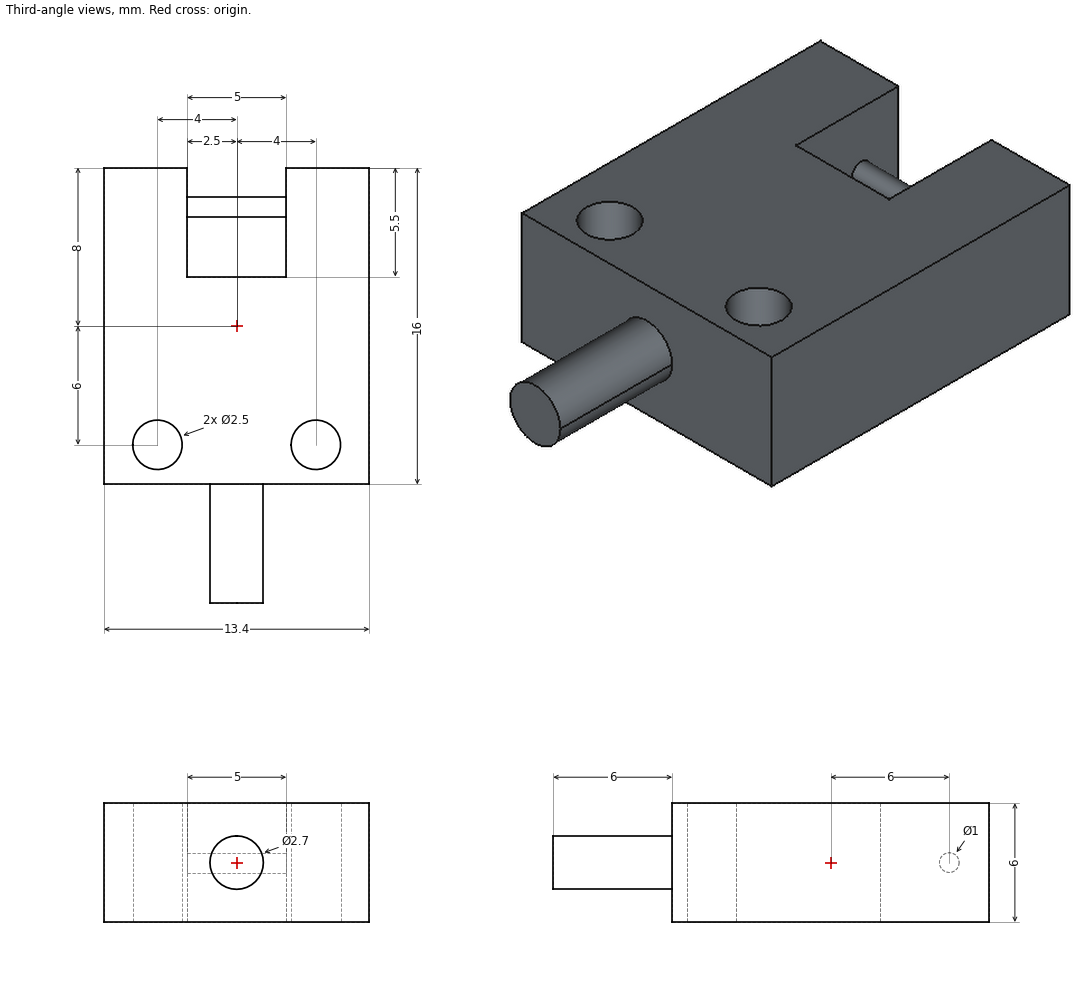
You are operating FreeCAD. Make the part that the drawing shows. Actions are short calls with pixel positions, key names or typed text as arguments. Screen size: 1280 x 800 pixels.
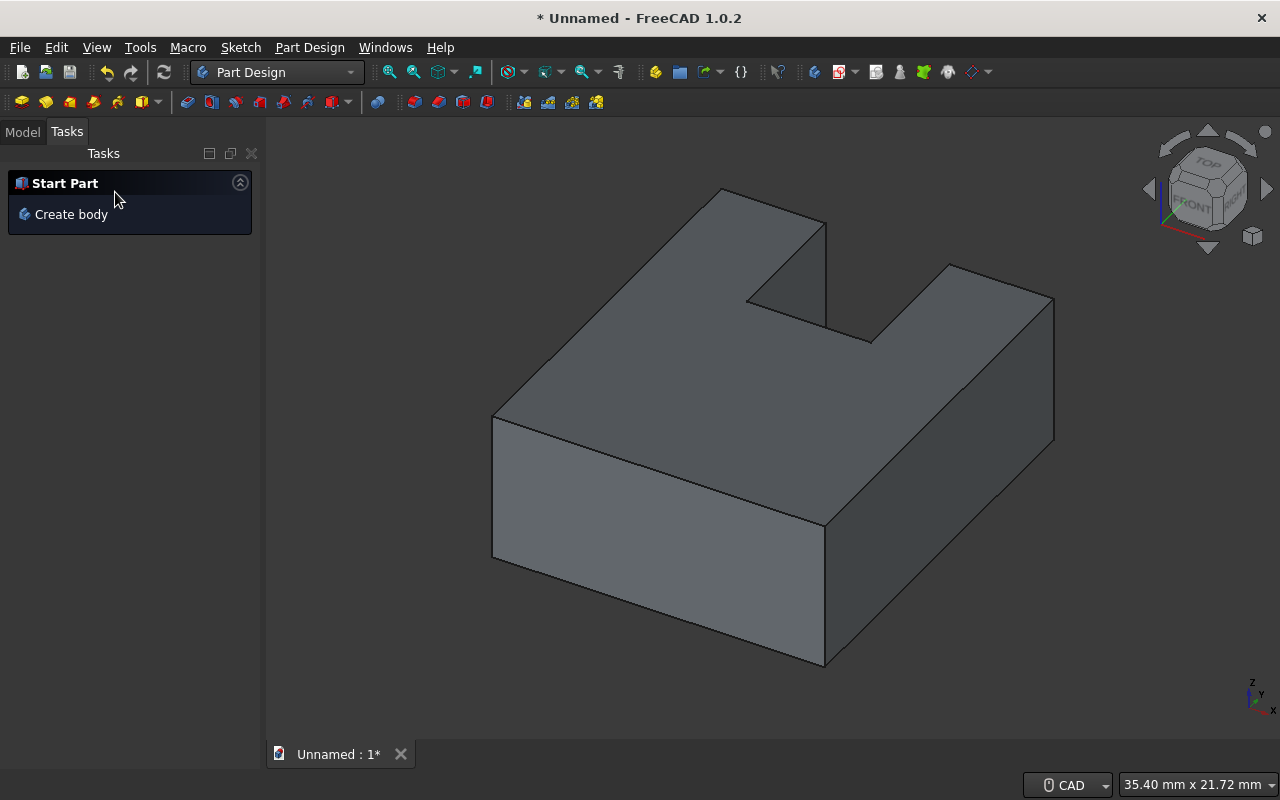
click(706, 557)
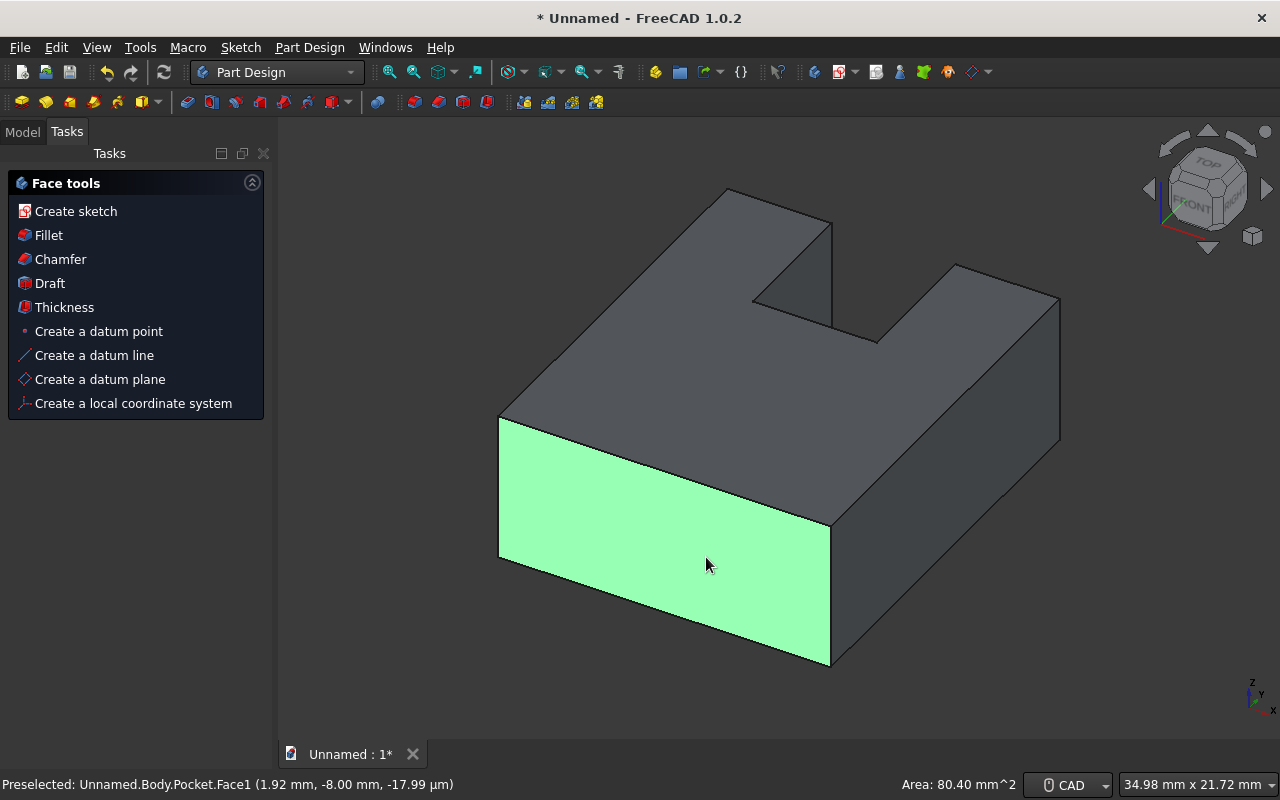
click(840, 72)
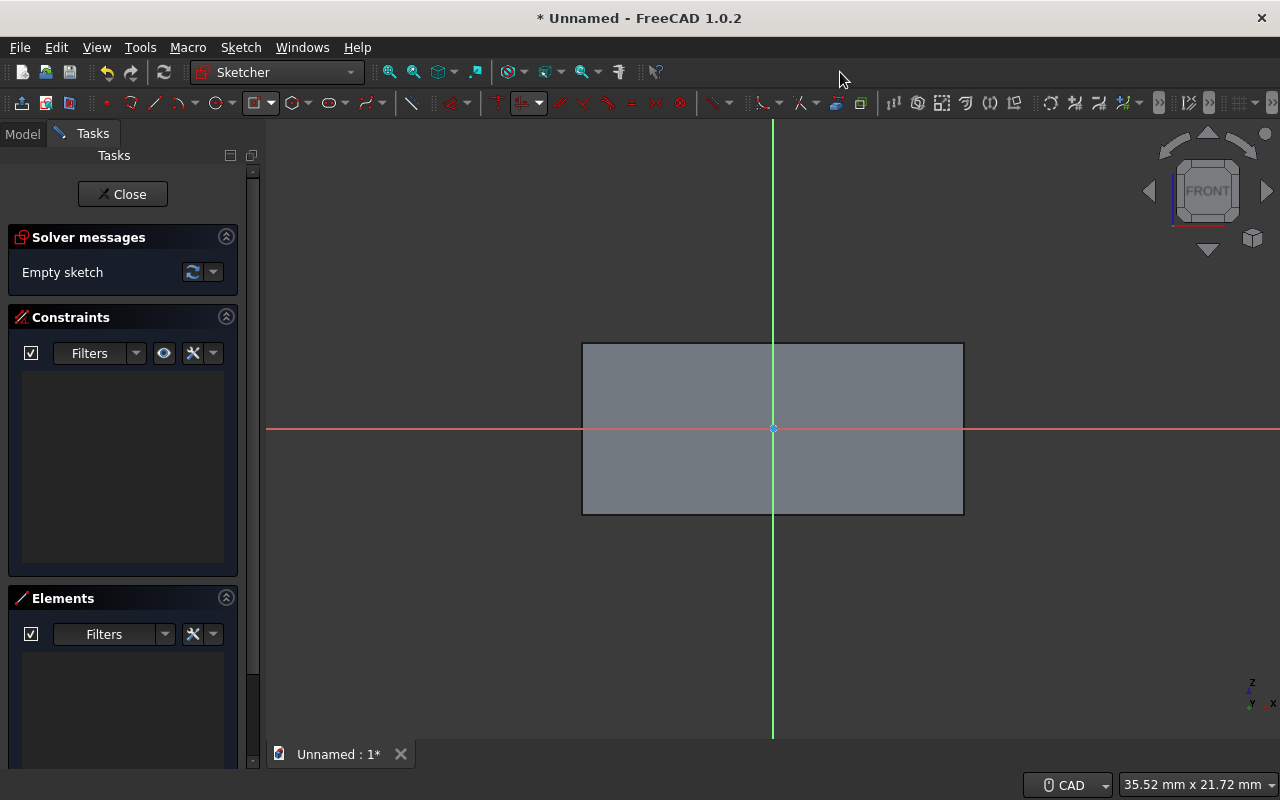
scroll(790, 429, up, 8)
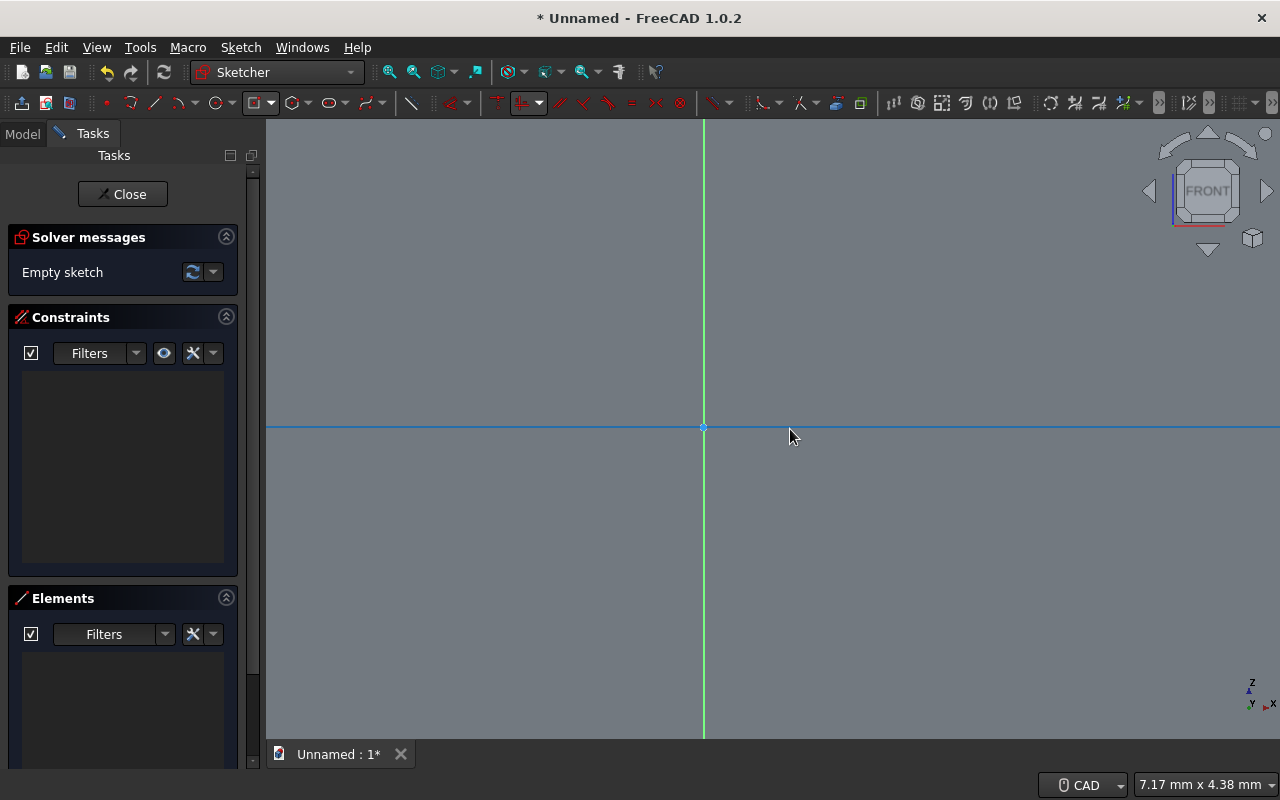
click(216, 104)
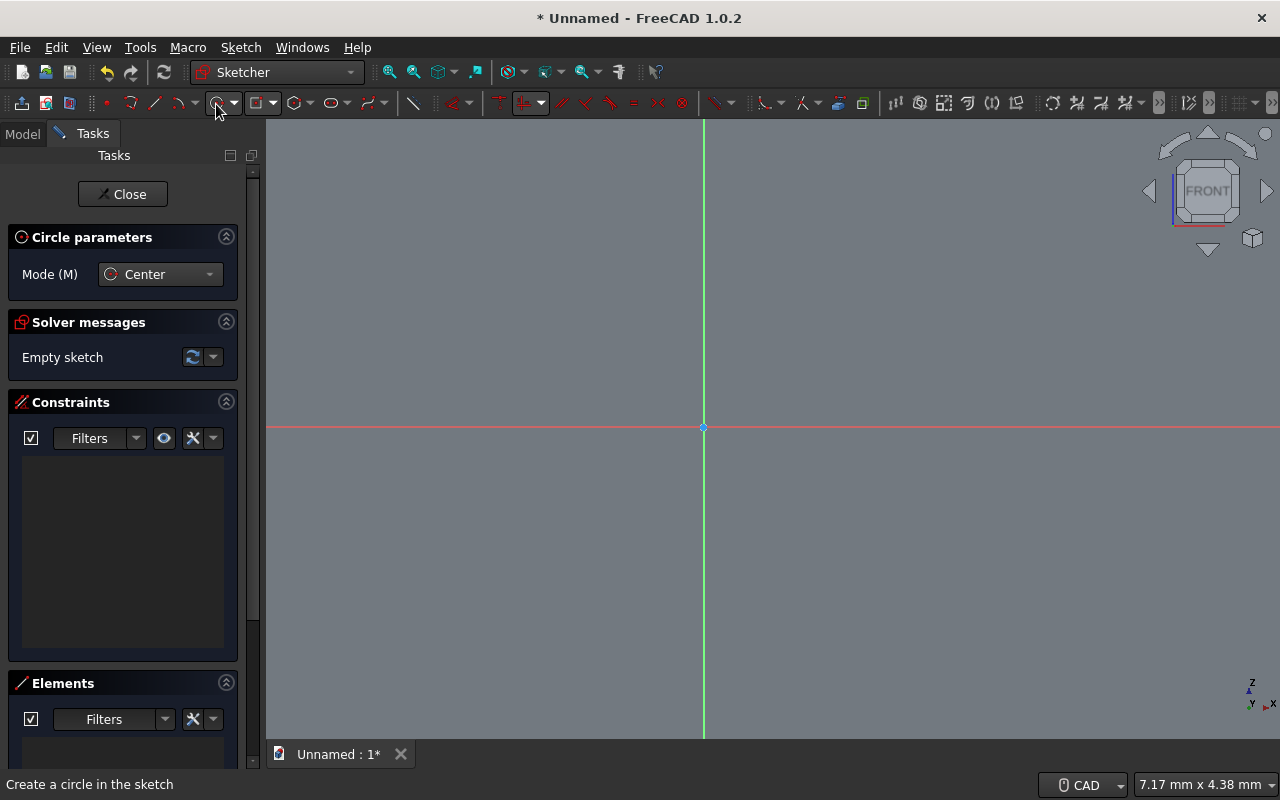
click(704, 427)
move(839, 292)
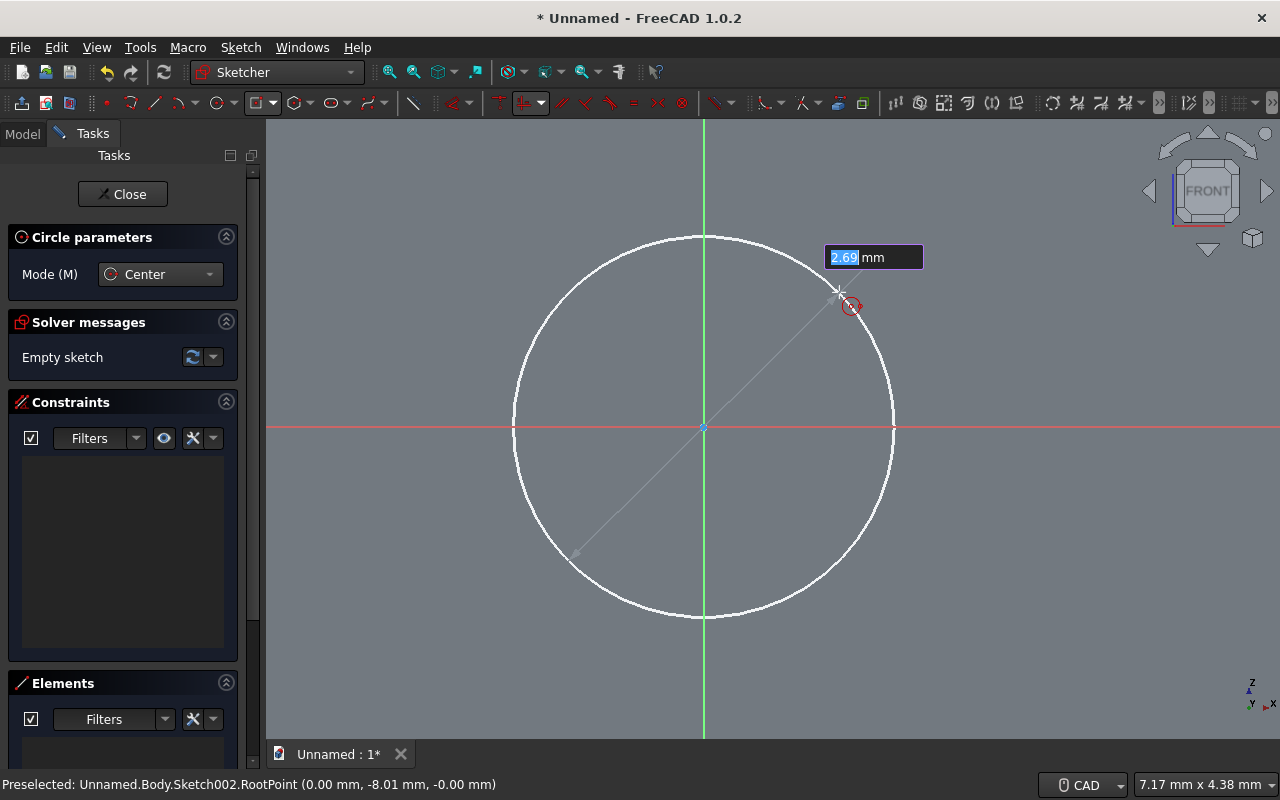
text(2.7)
key(Return)
key(Escape)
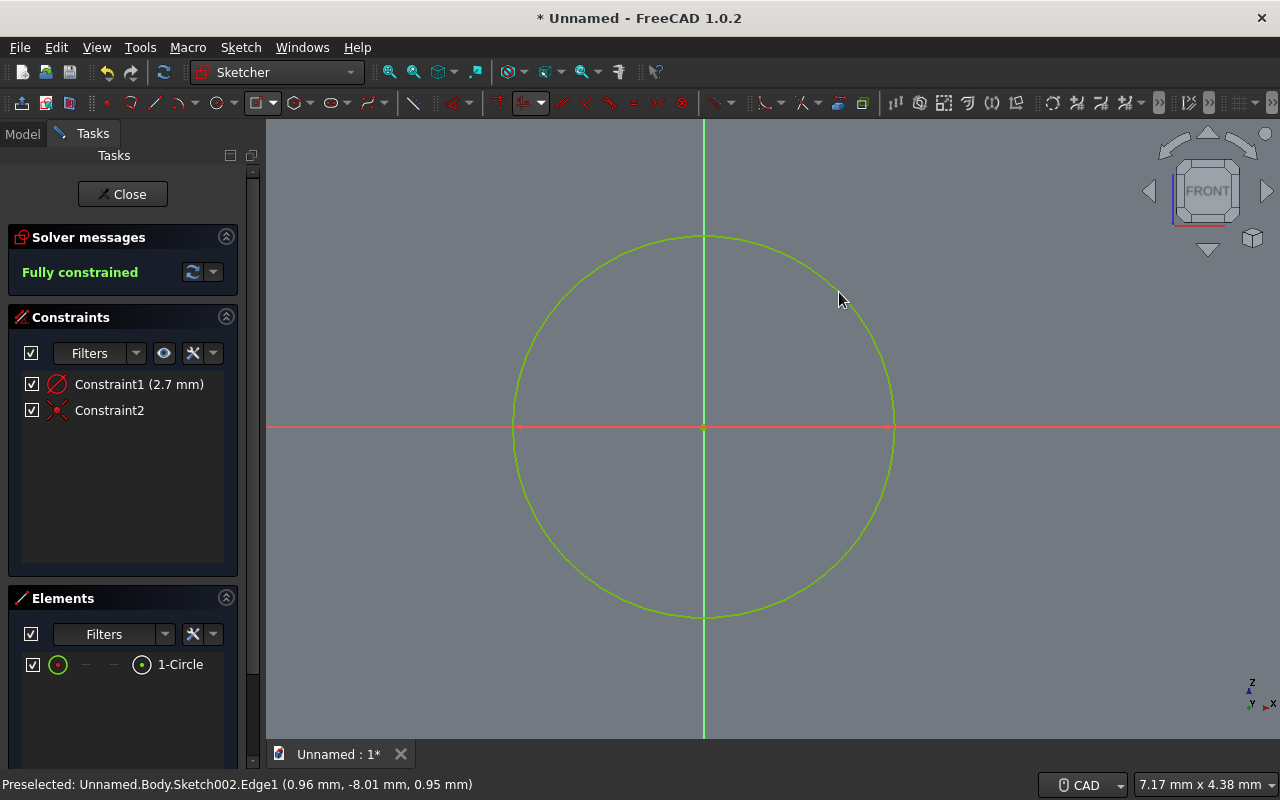
click(123, 194)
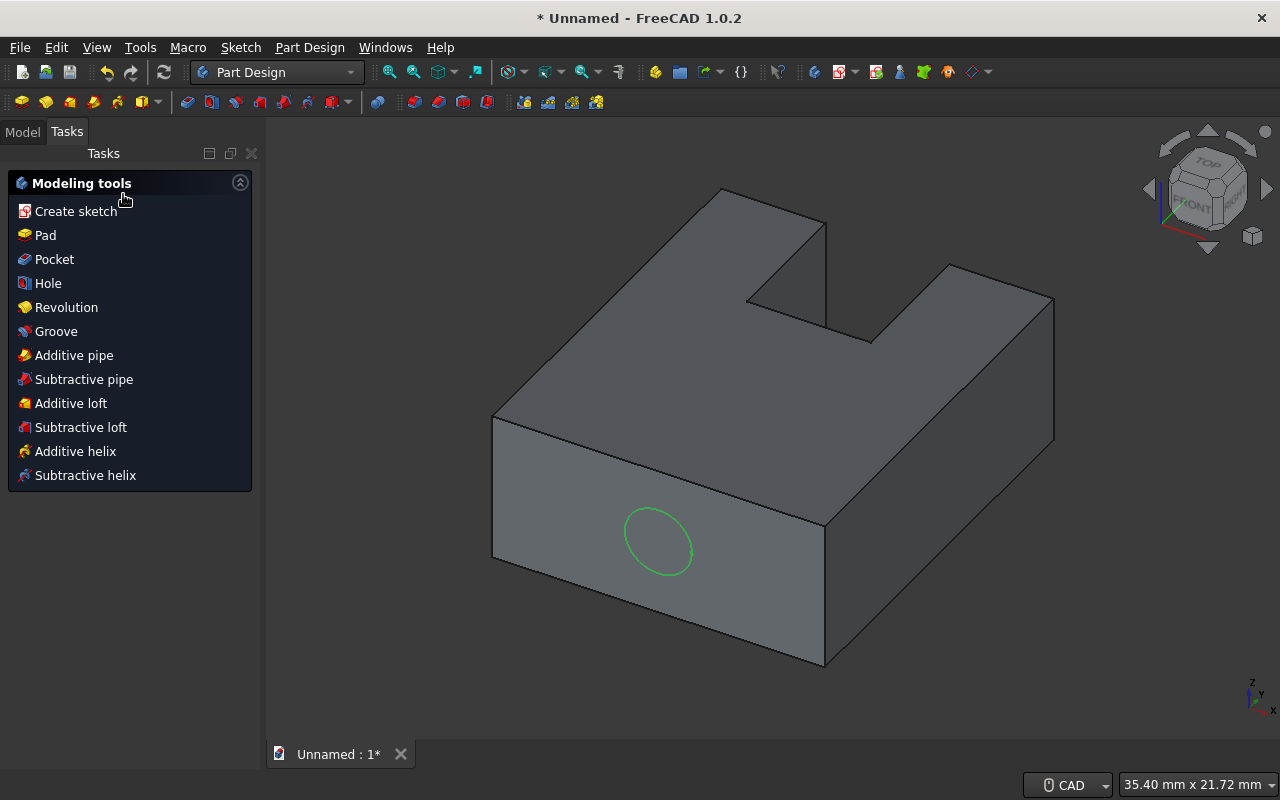
click(22, 102)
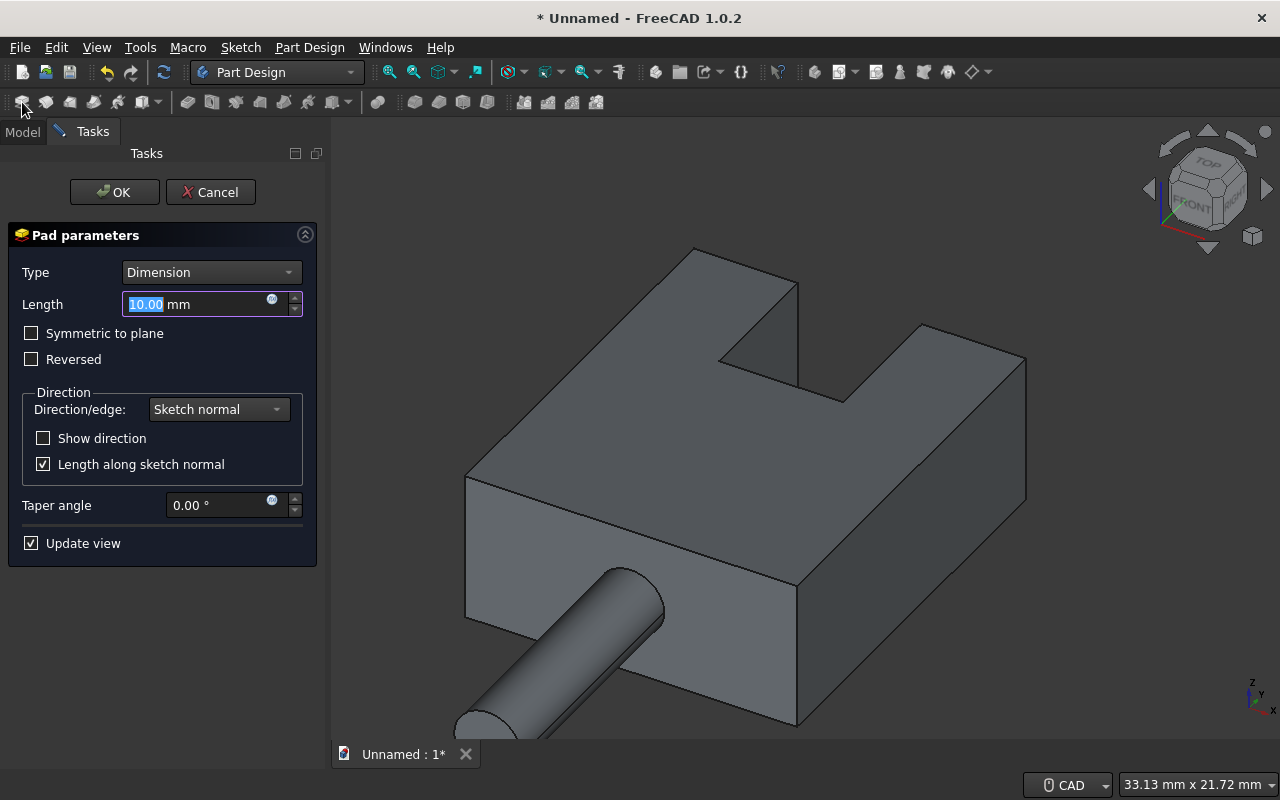
text(6)
key(Tab)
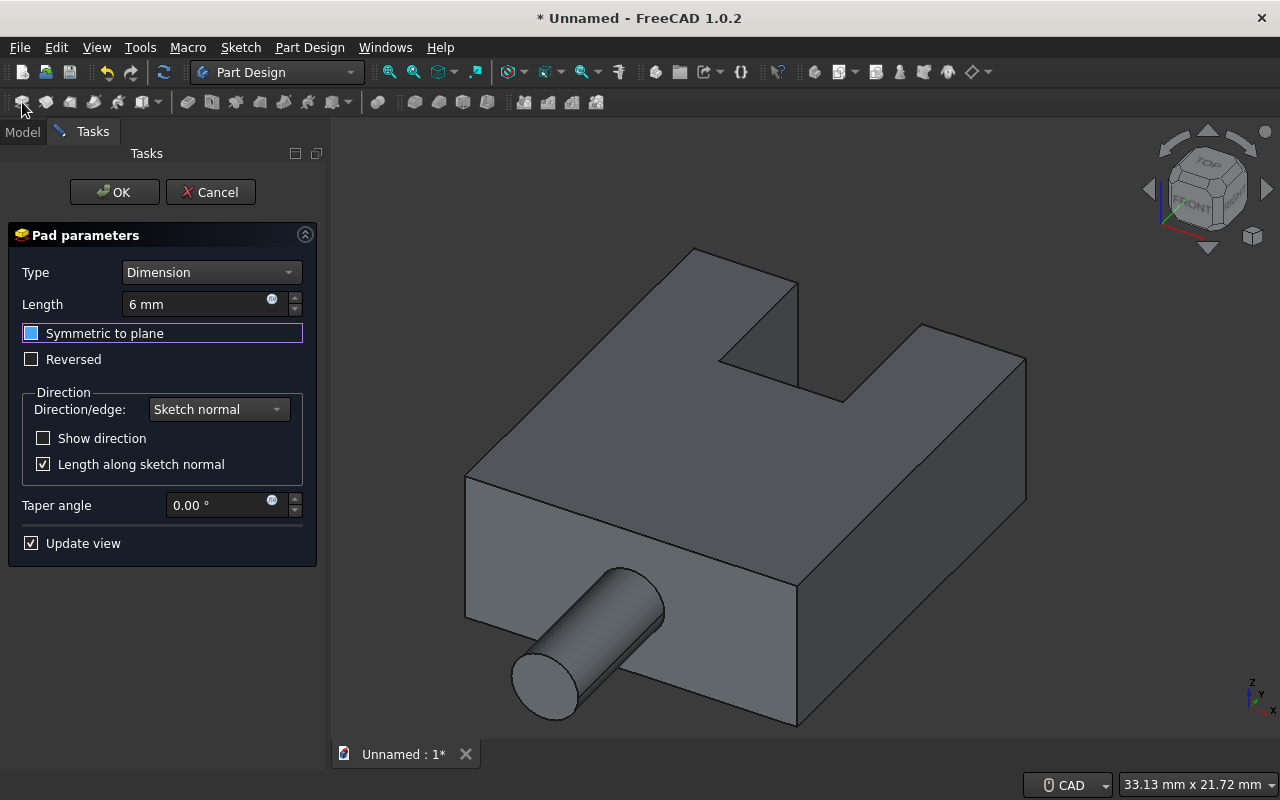
click(115, 192)